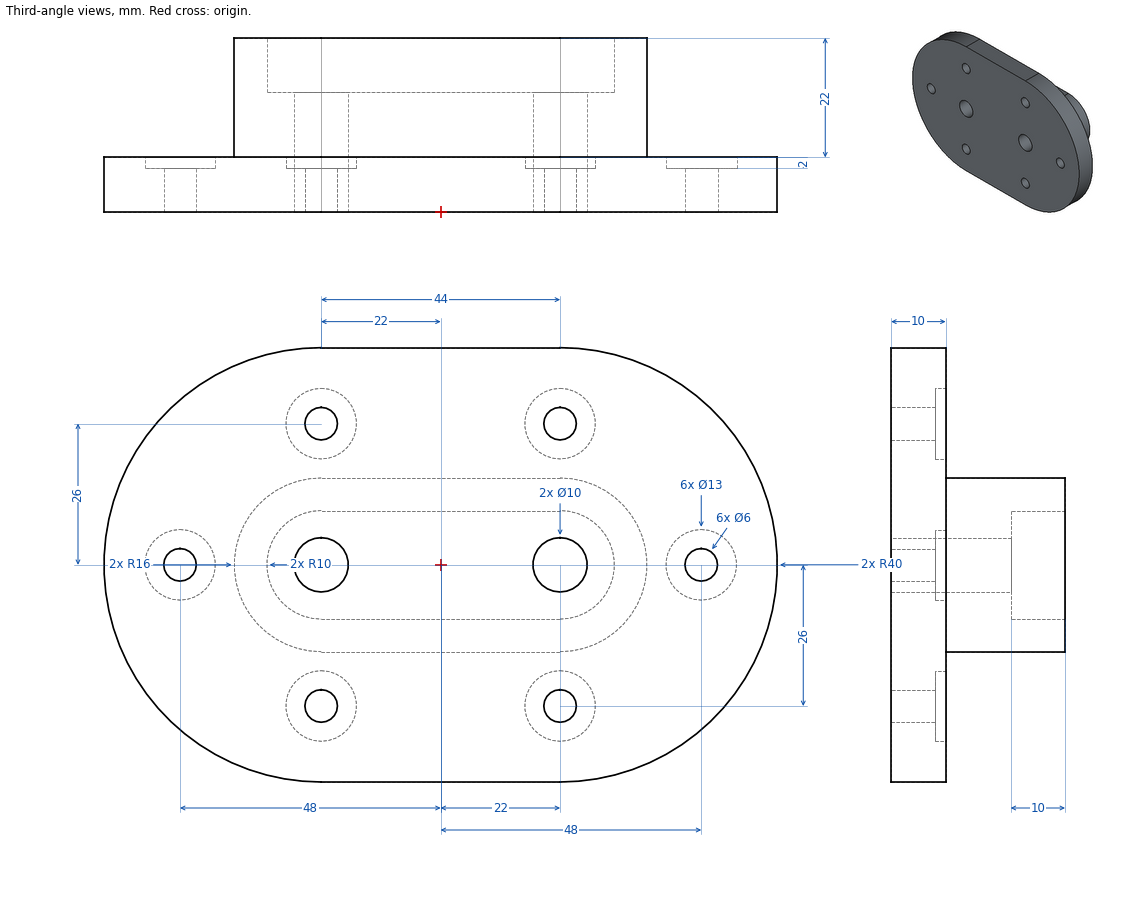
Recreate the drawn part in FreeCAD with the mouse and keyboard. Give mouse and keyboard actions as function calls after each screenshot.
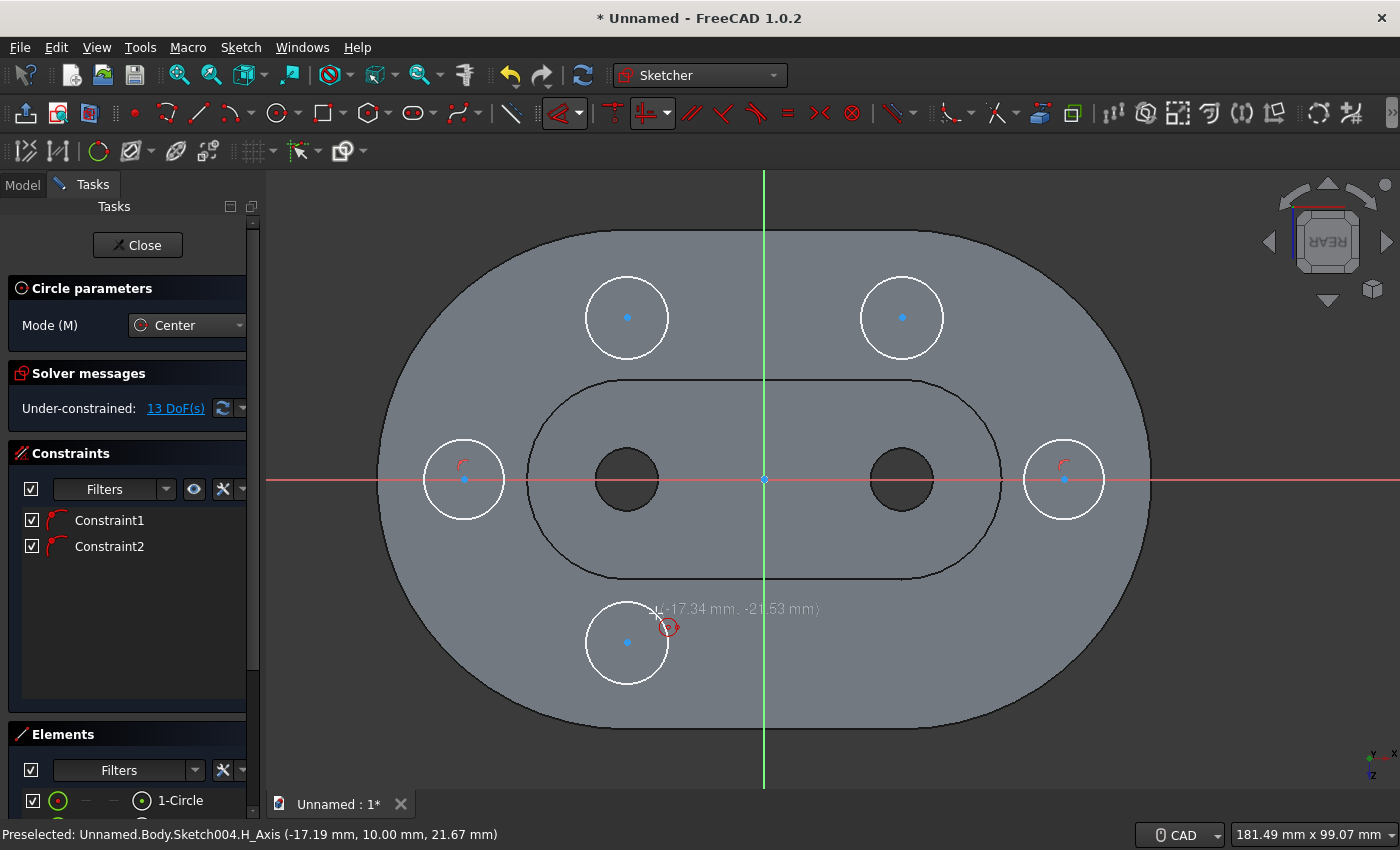
click(902, 642)
click(931, 613)
key(Escape)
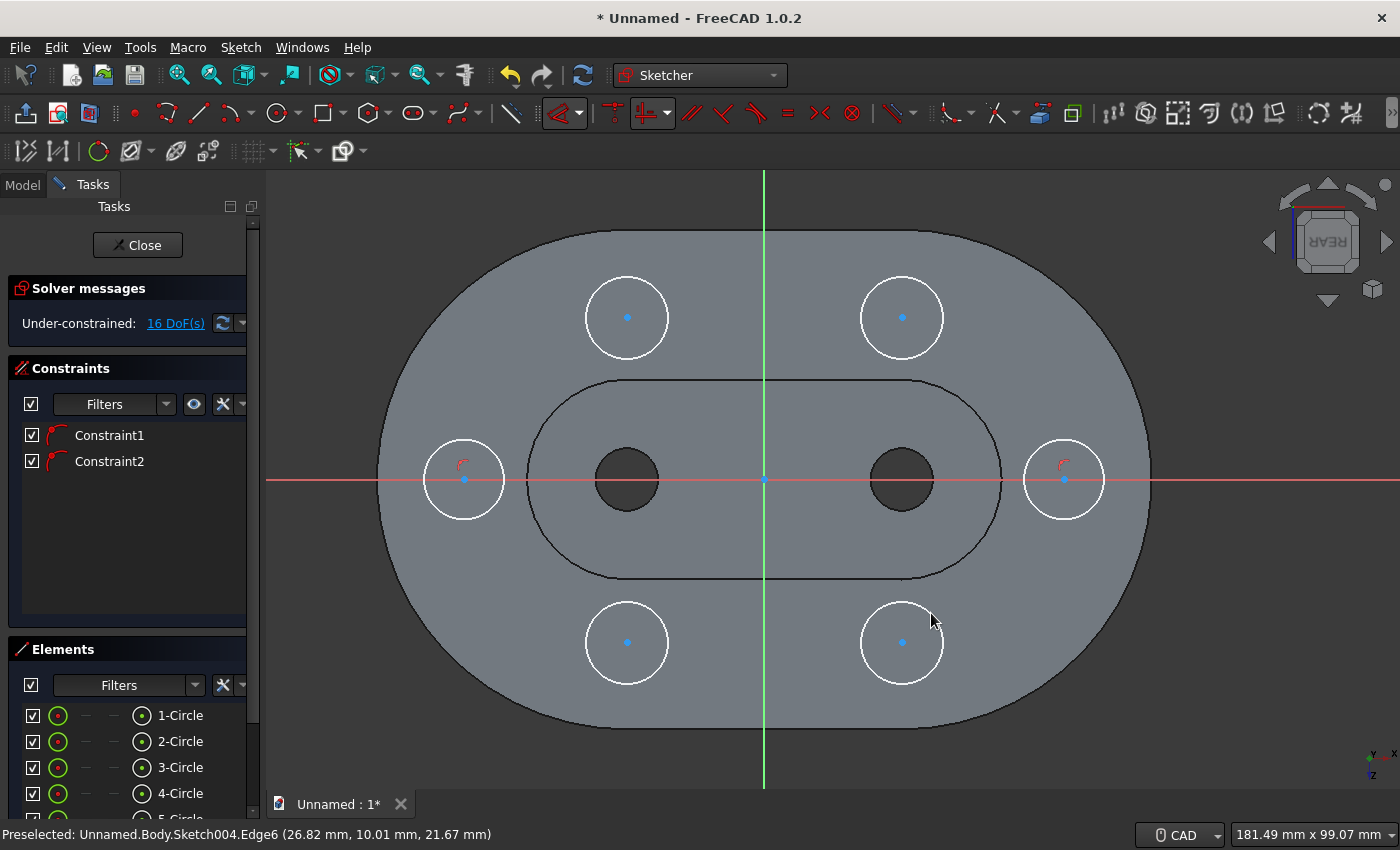
click(1092, 451)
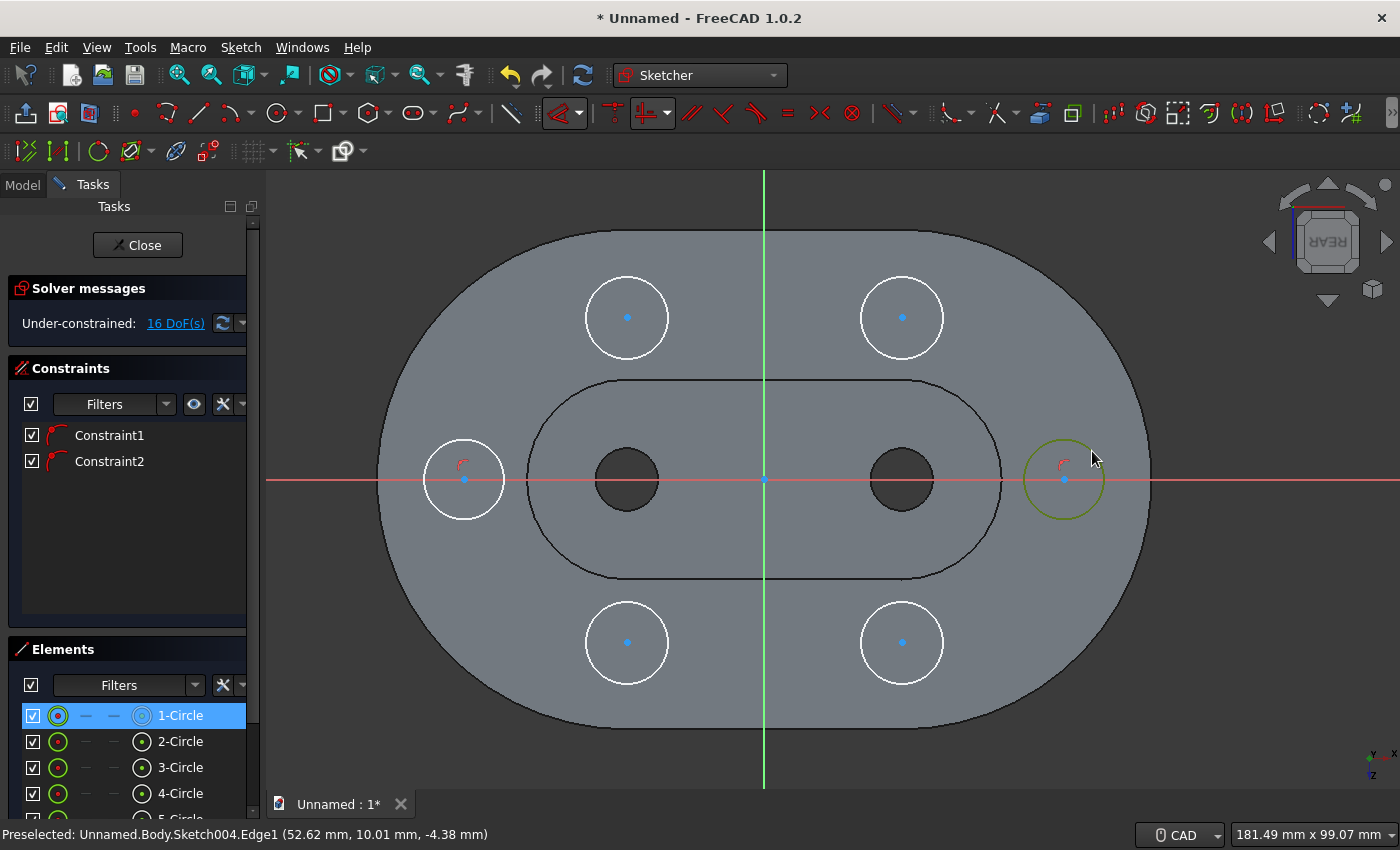
click(931, 289)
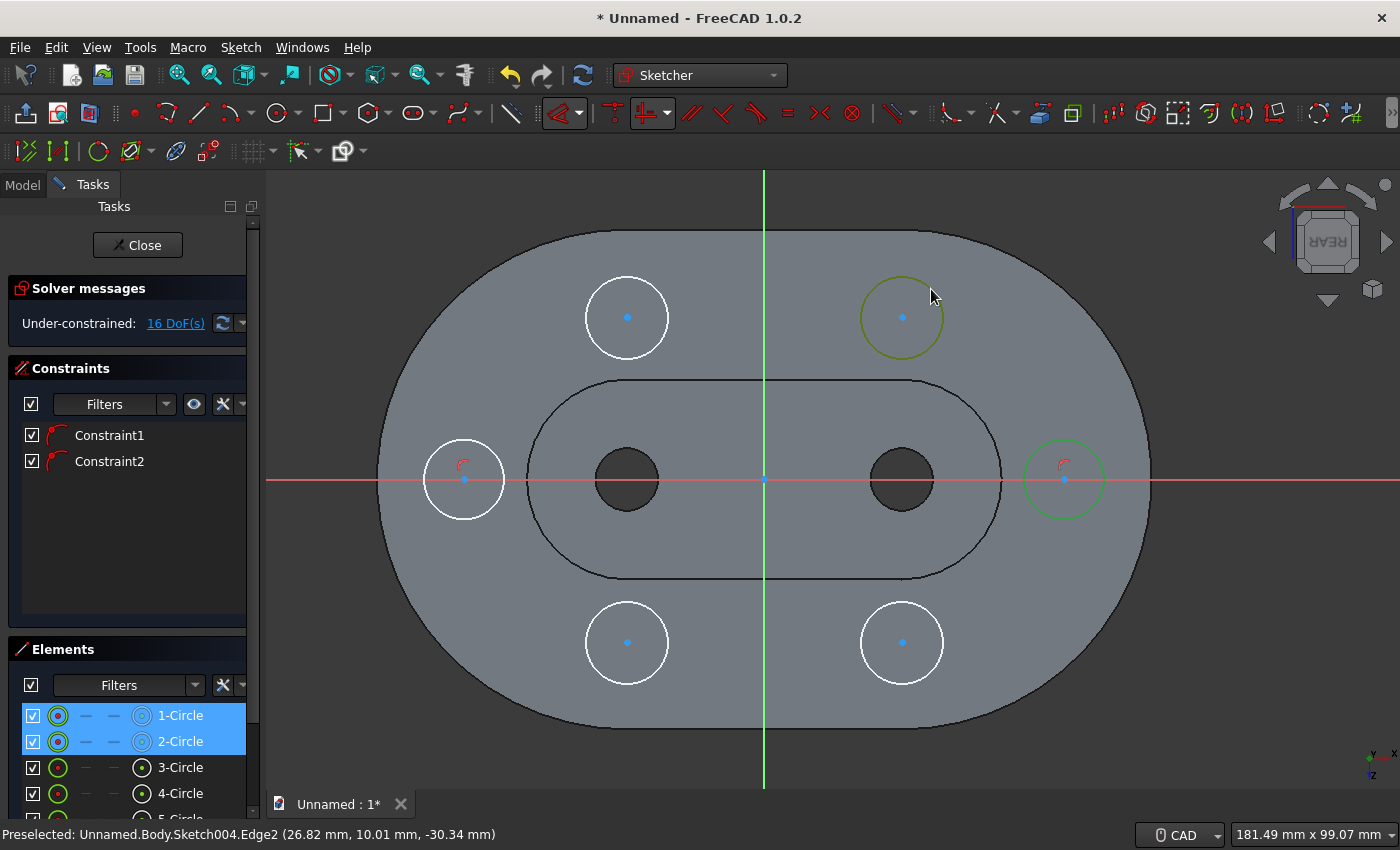
click(656, 289)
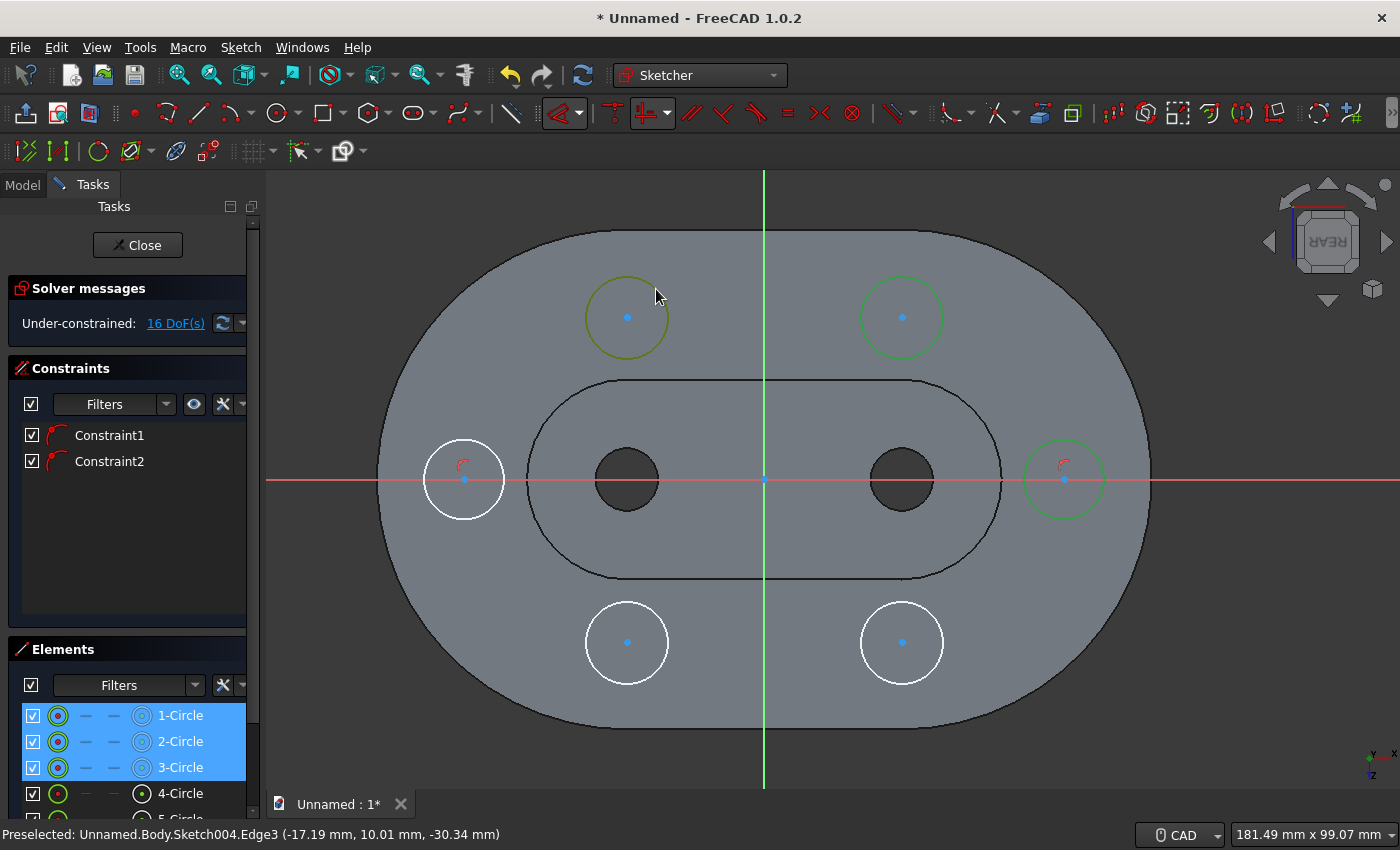
click(492, 451)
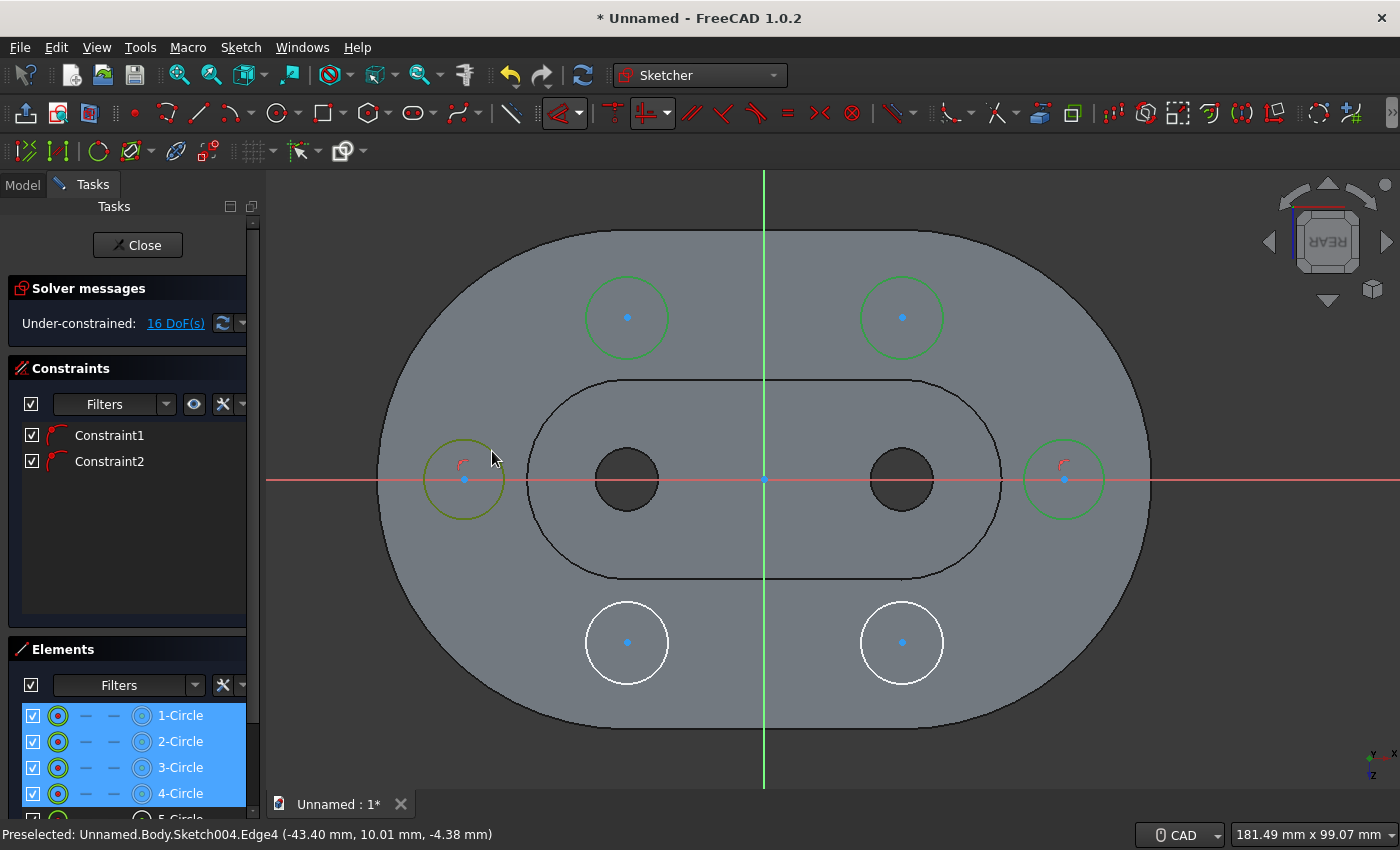
click(656, 614)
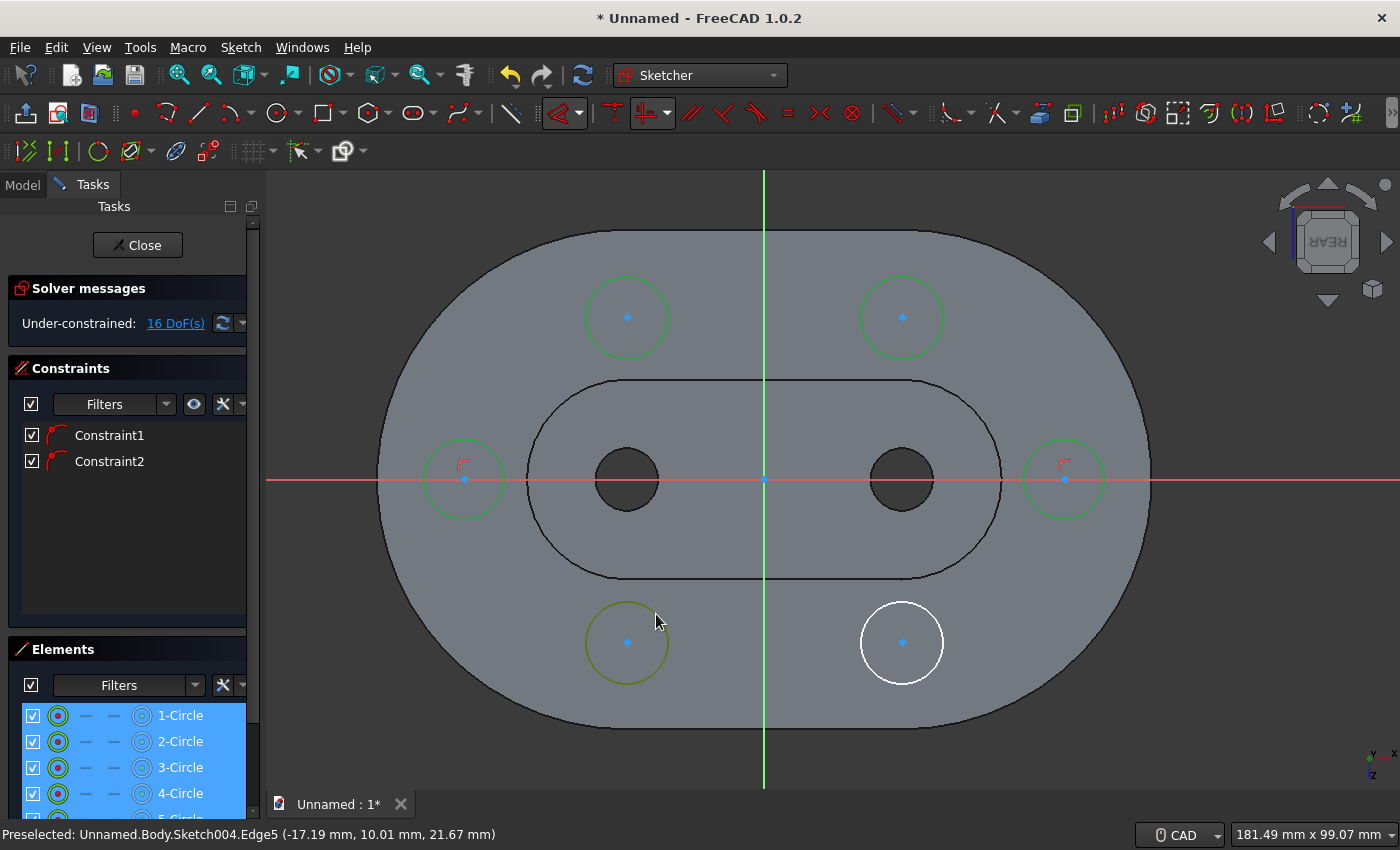
click(931, 614)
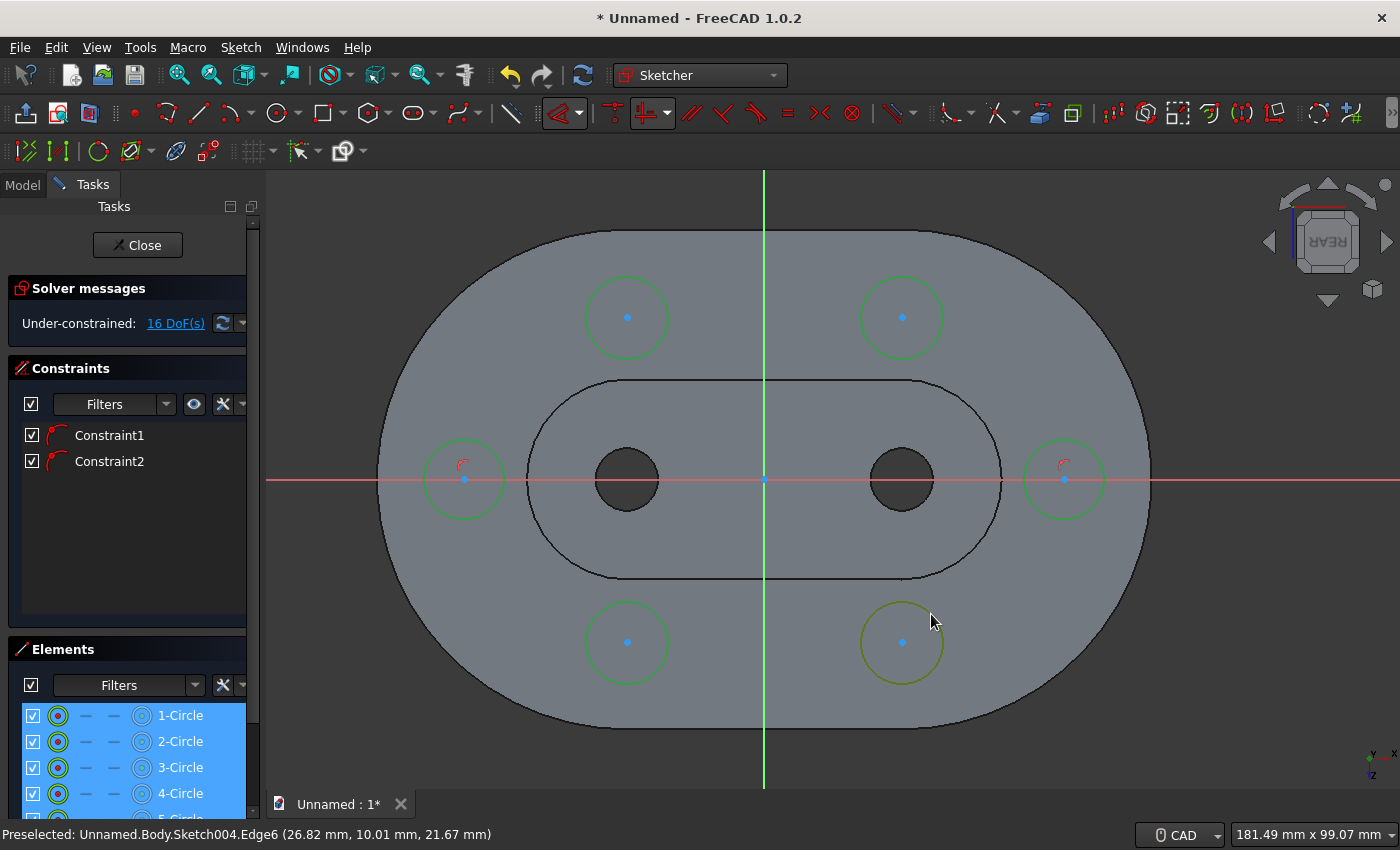
click(788, 114)